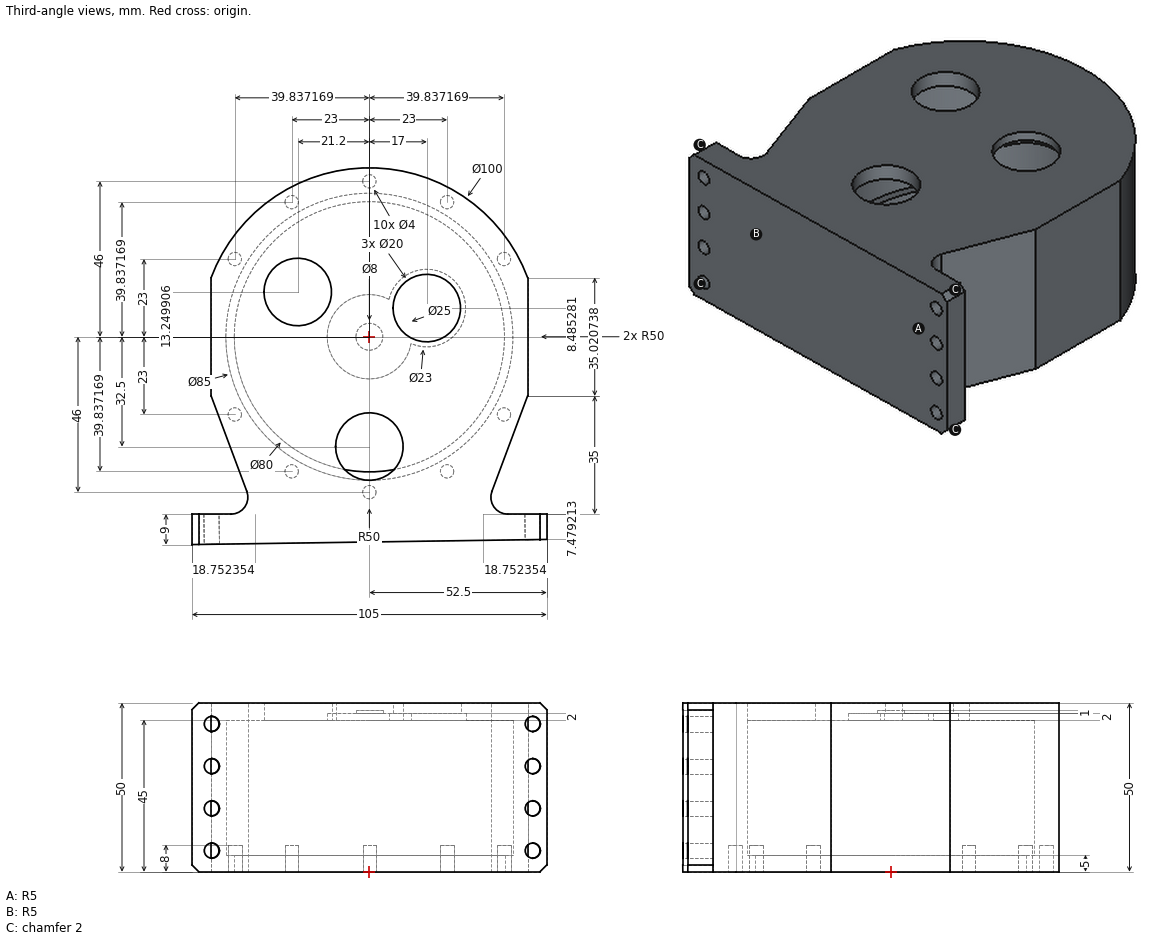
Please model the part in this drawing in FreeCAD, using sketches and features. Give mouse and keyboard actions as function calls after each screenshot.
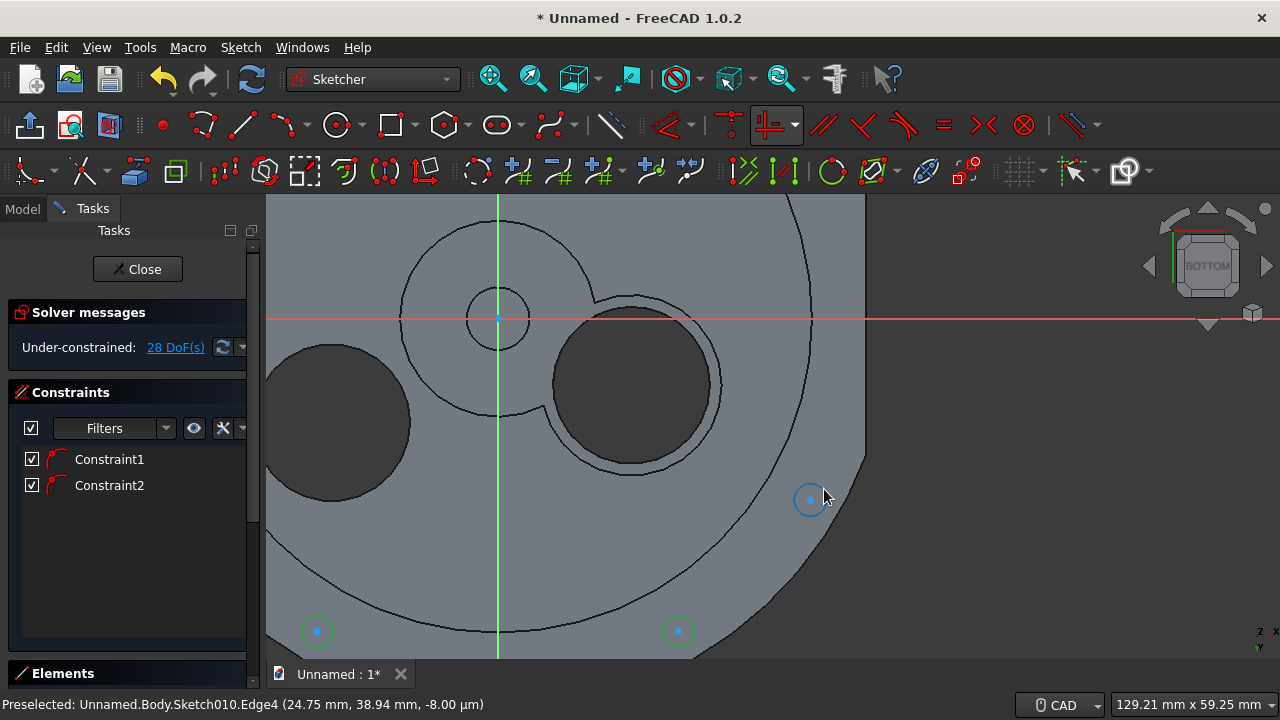
click(822, 489)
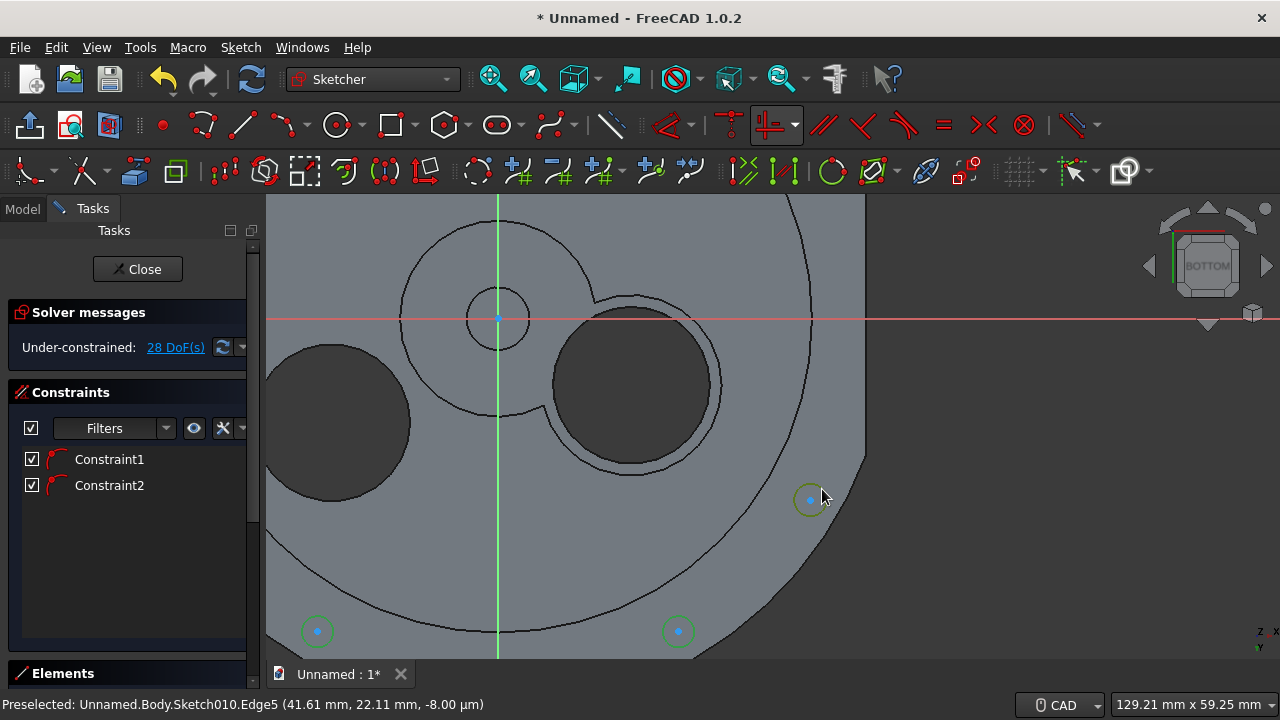
scroll(825, 489, down, 5)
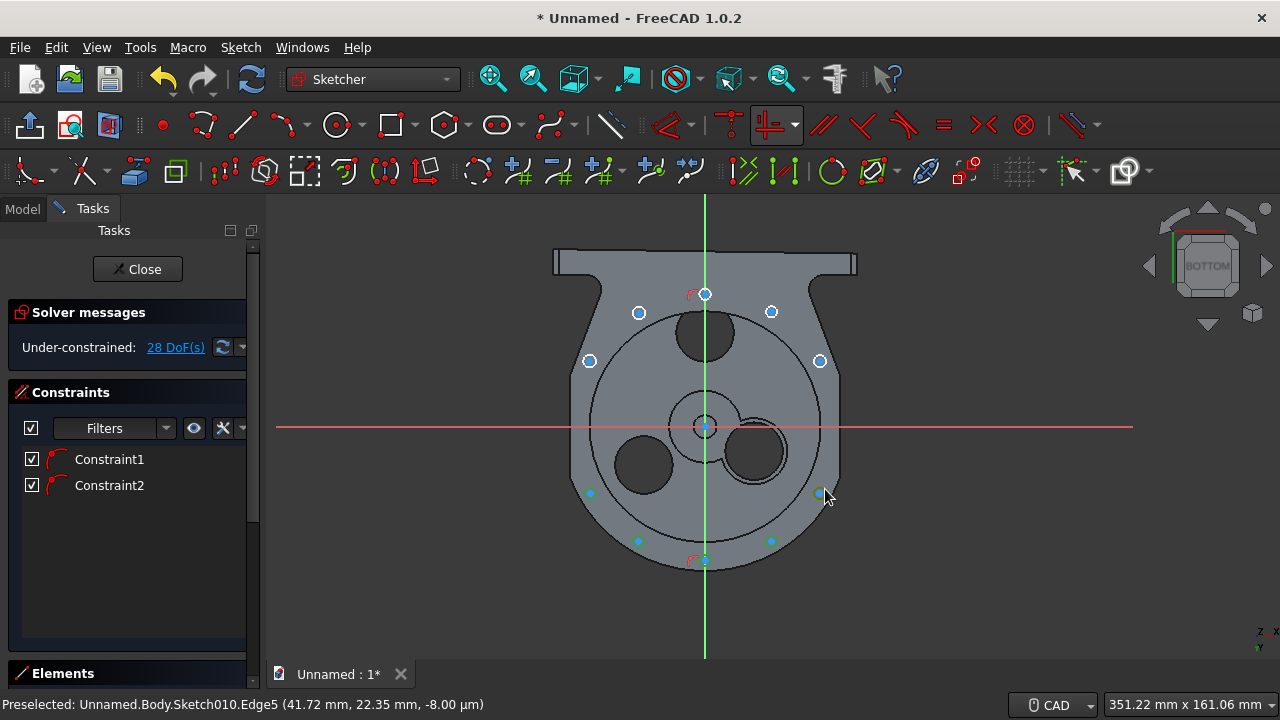
scroll(594, 357, up, 4)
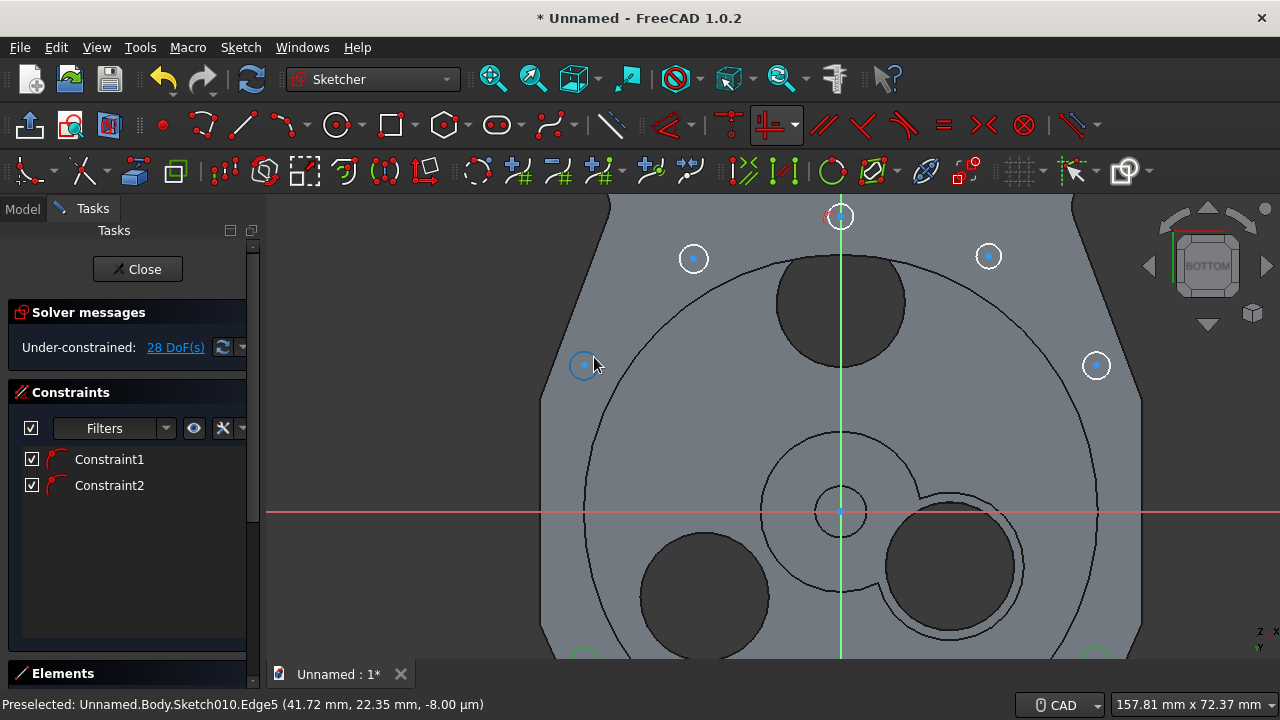
click(594, 356)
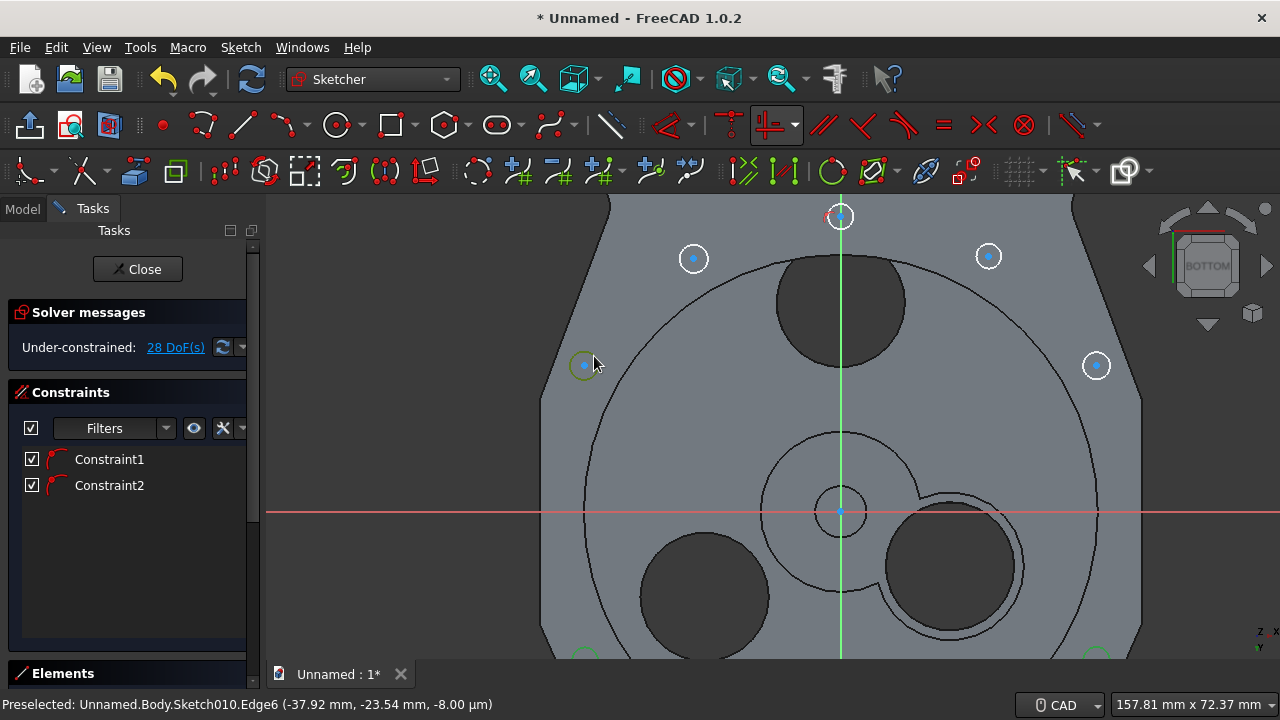
click(704, 249)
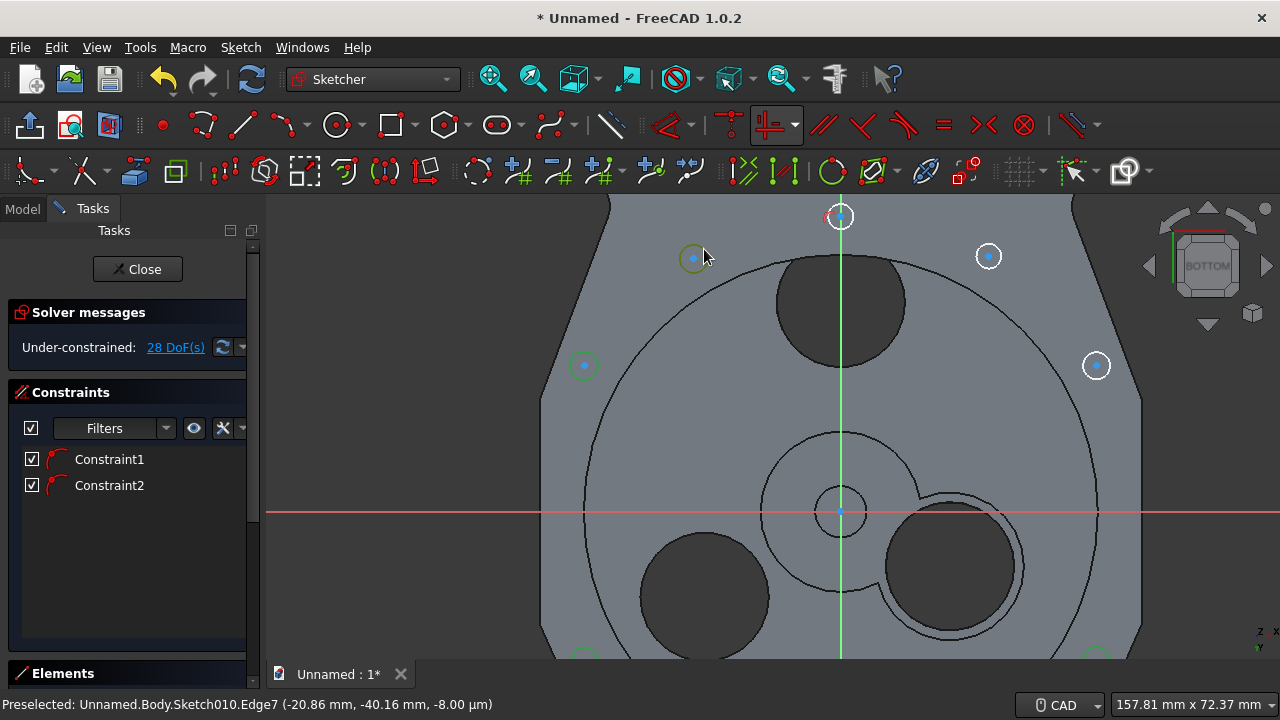
click(840, 229)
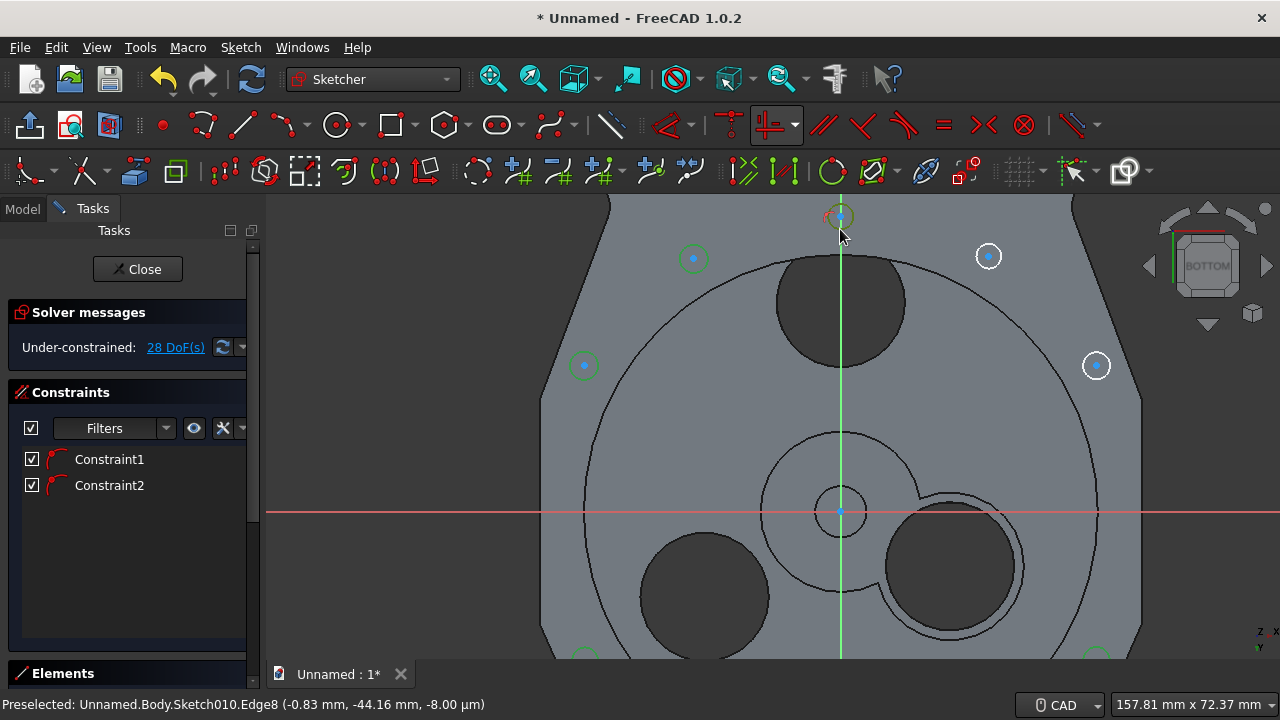
click(997, 247)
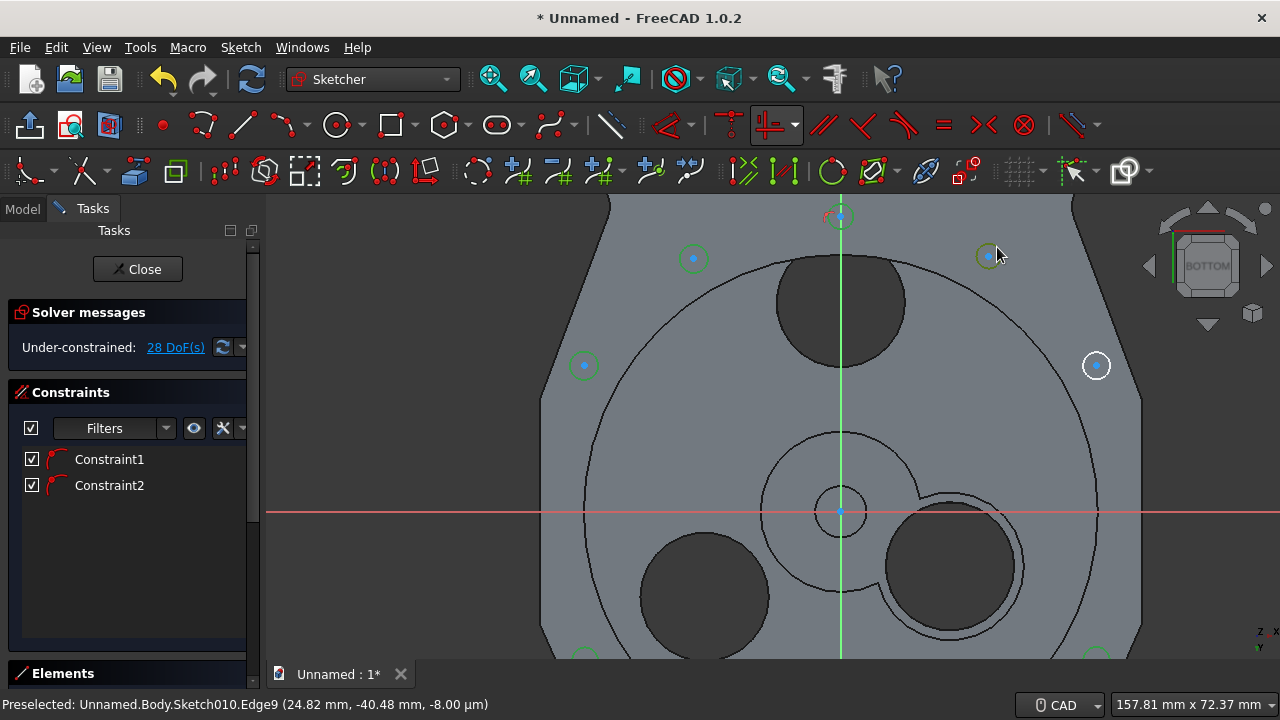
click(1106, 356)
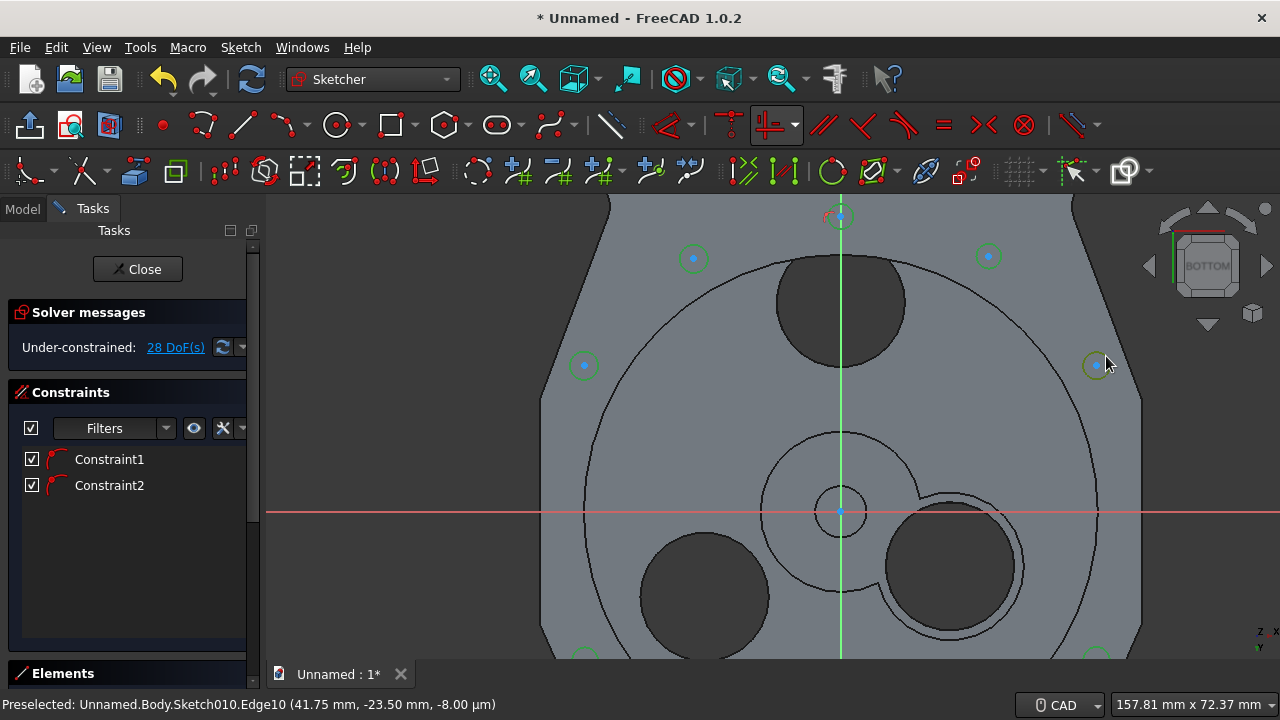
click(944, 126)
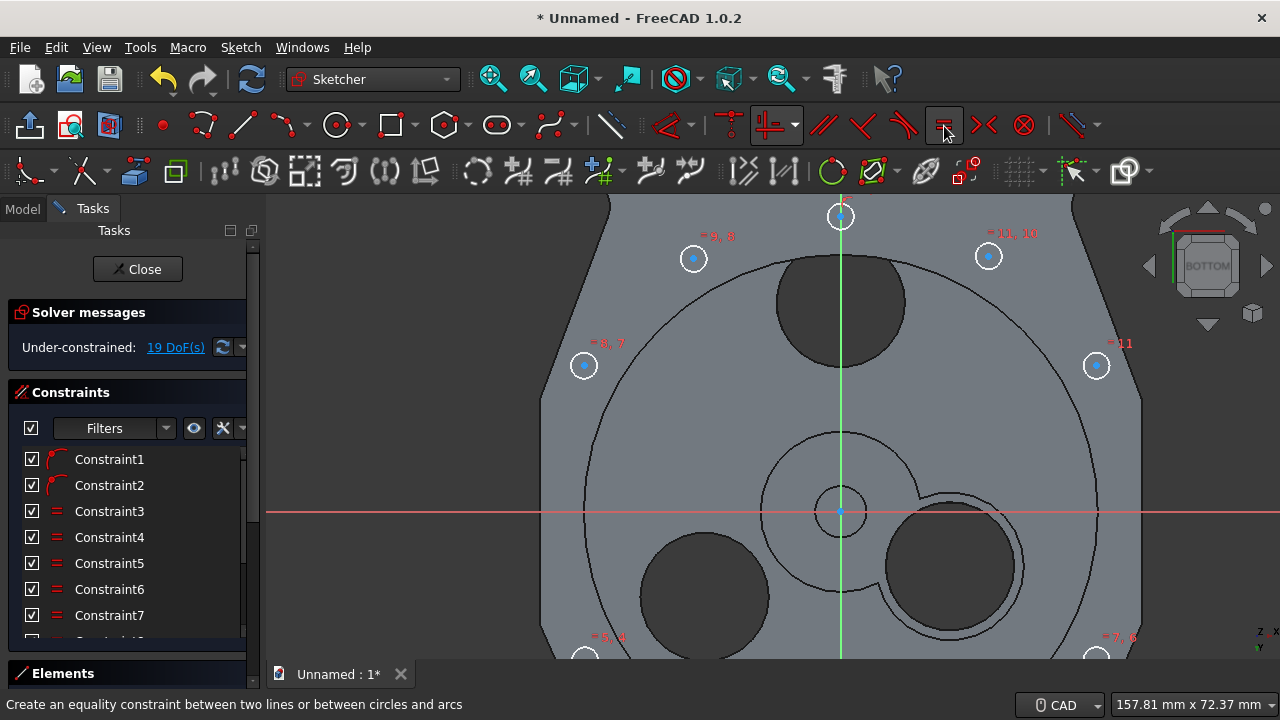
scroll(593, 357, down, 4)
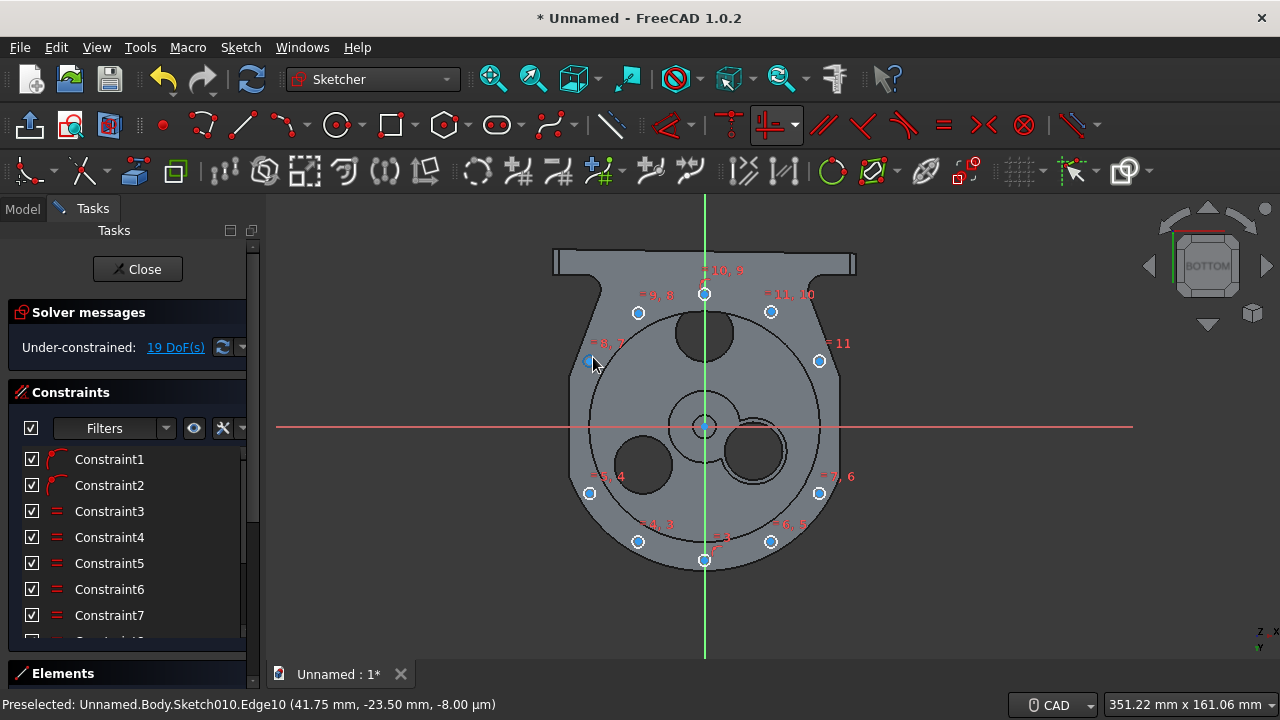
click(638, 542)